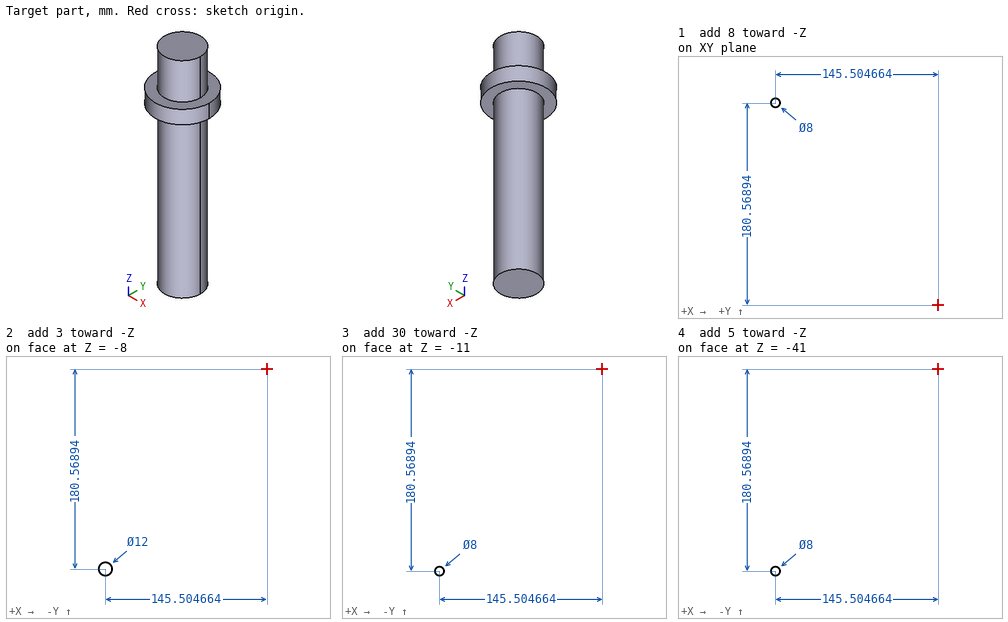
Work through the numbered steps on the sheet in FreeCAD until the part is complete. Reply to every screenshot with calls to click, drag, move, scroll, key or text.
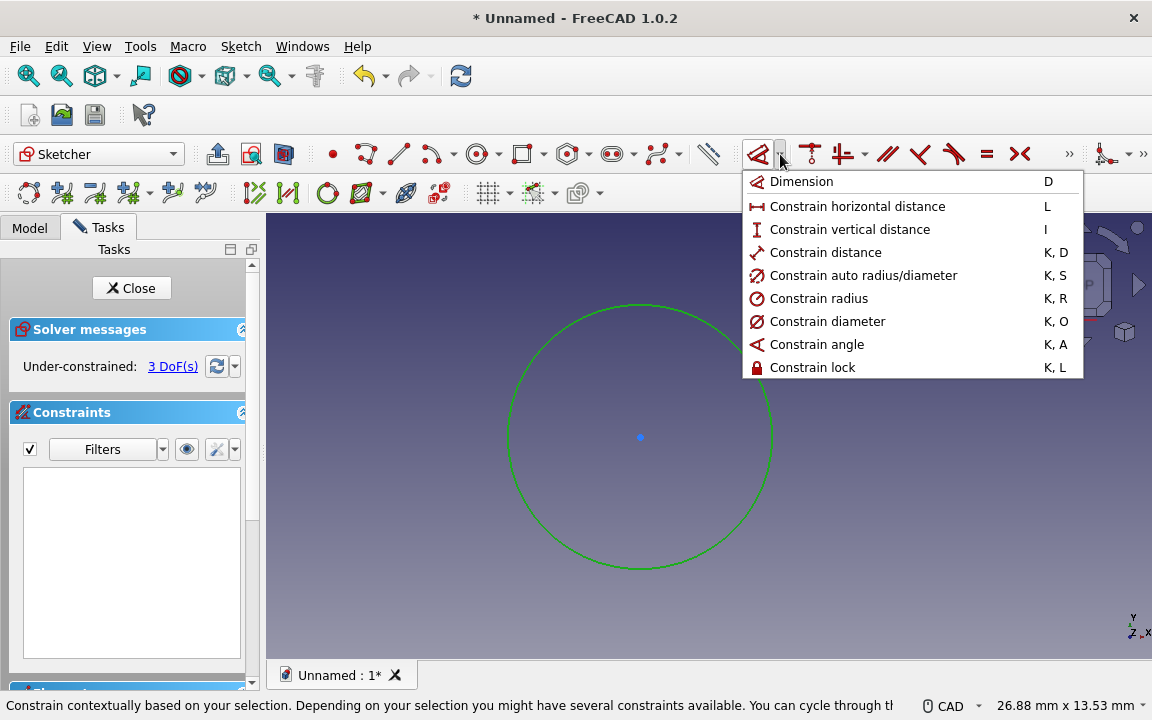
click(913, 322)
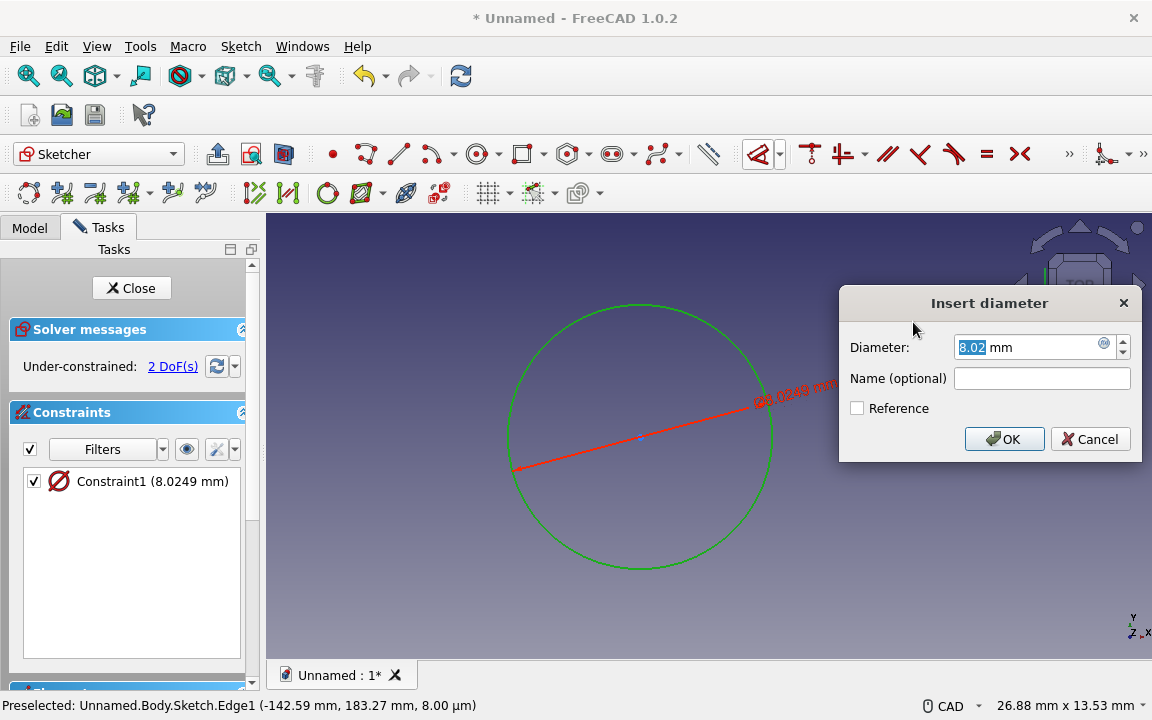
text(8)
key(Return)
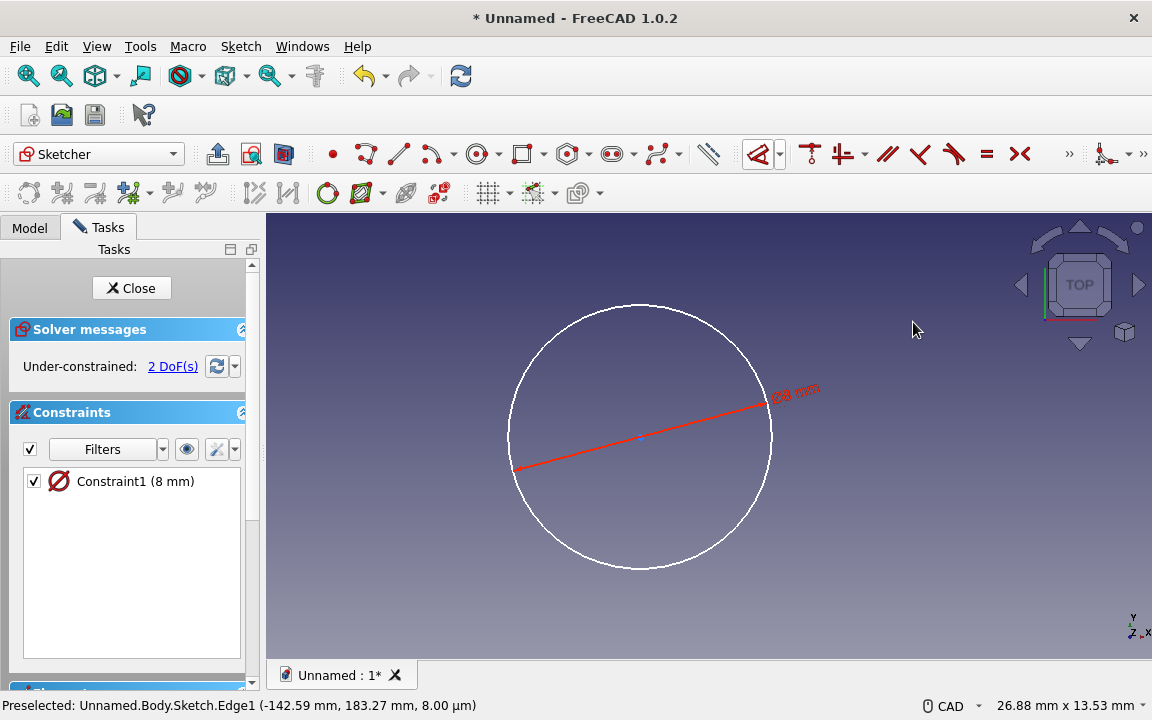
click(640, 437)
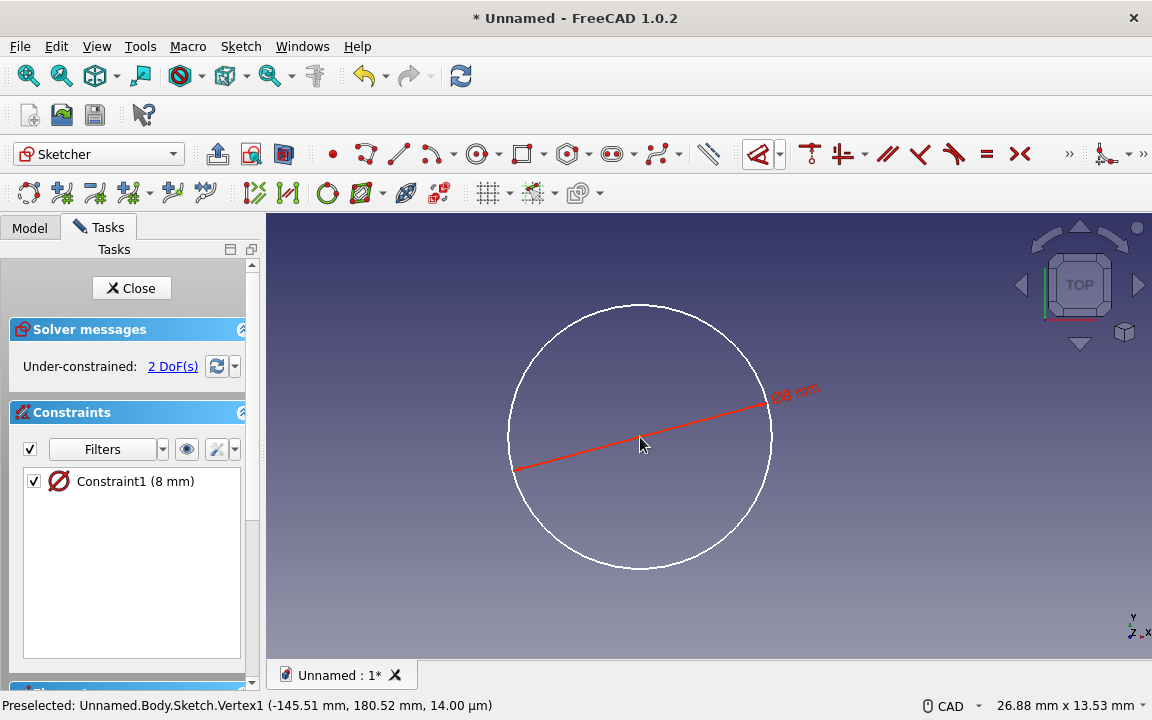
key(i)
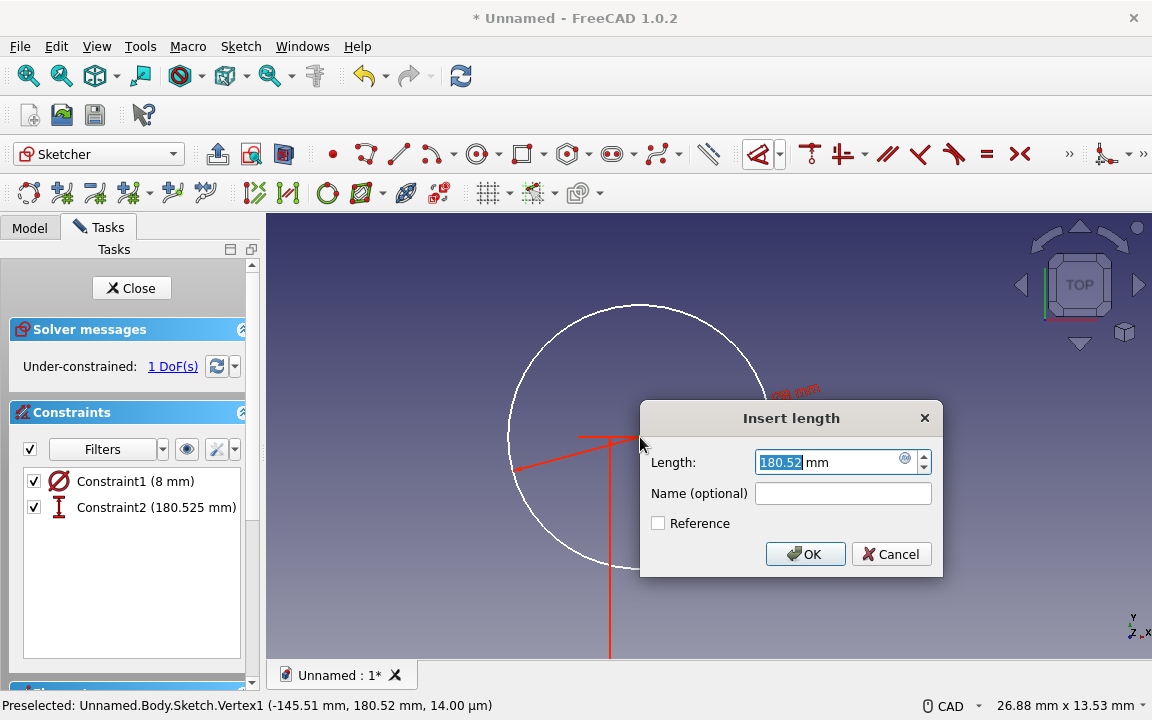
text(180.56894)
key(Return)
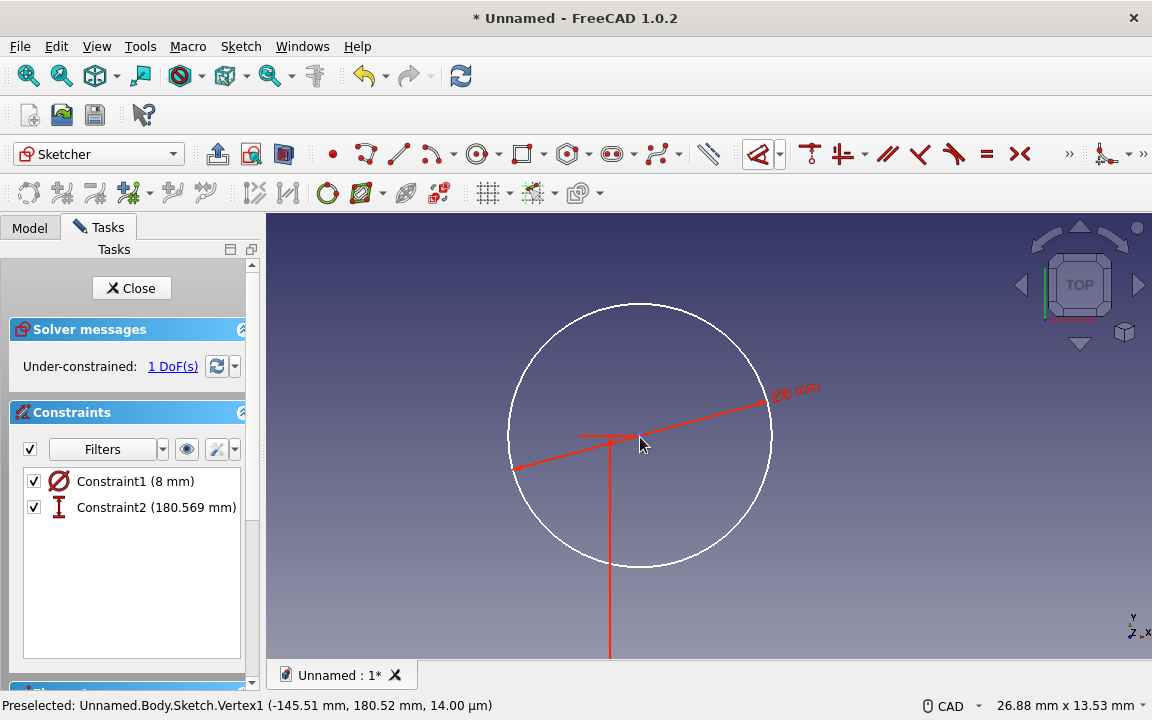
click(640, 436)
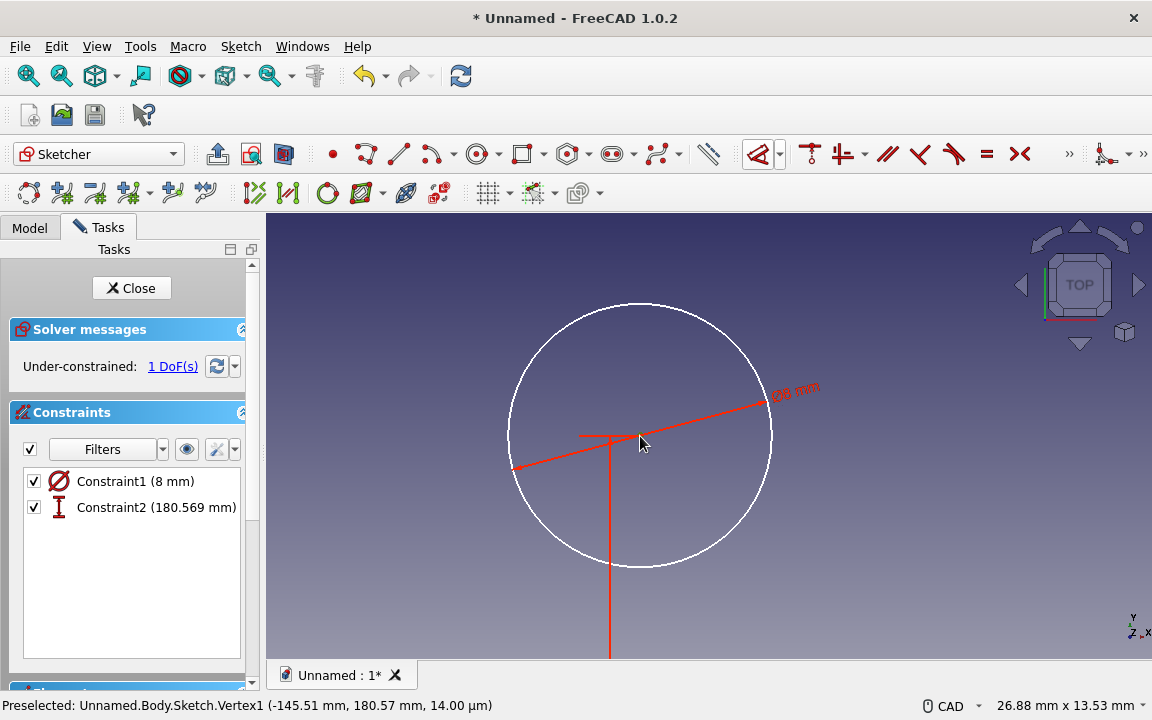
key(l)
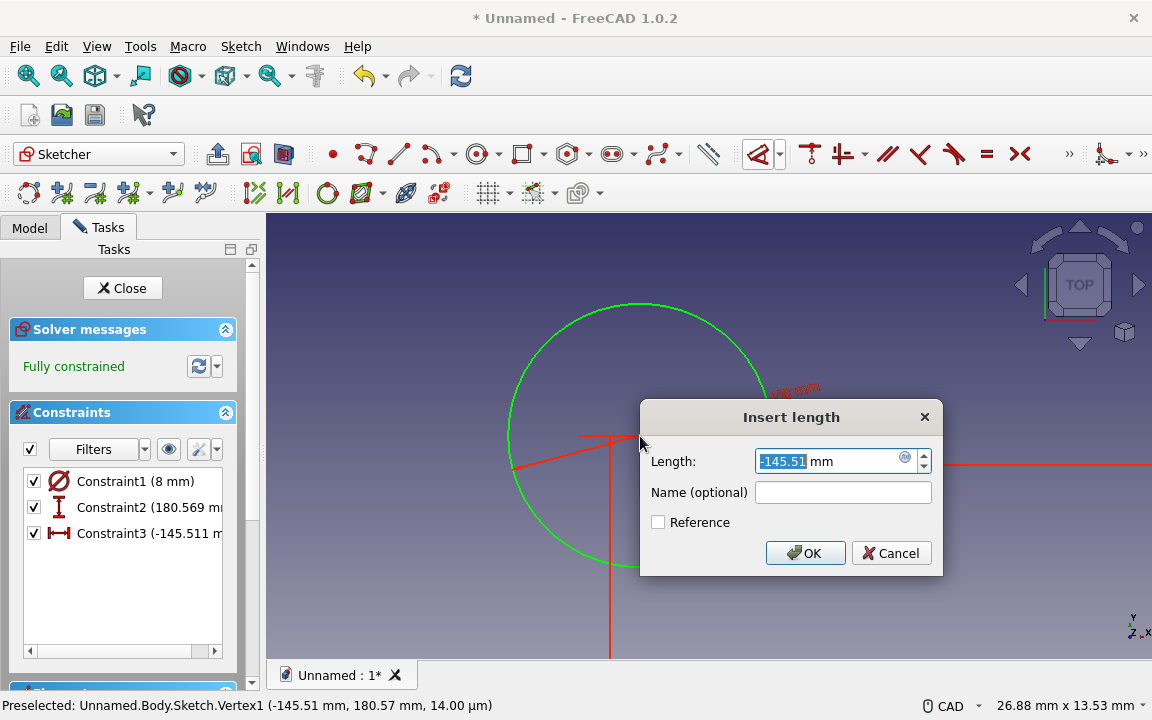
text(-145.504664)
key(Return)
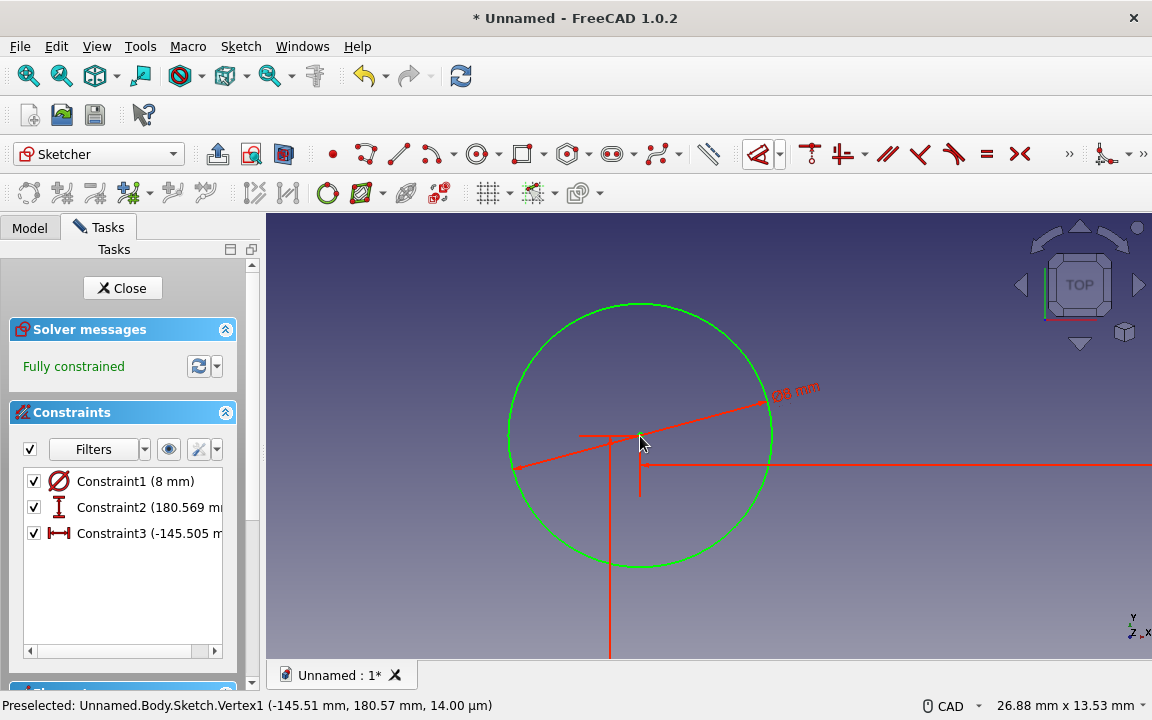
click(123, 288)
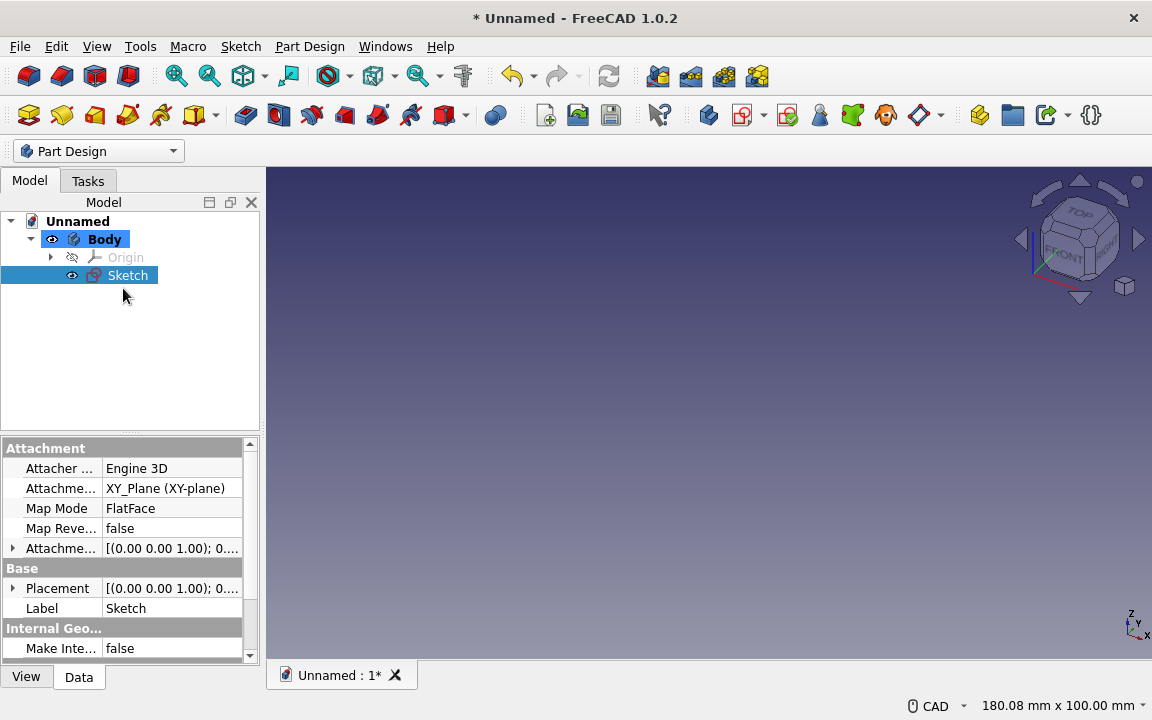
click(29, 116)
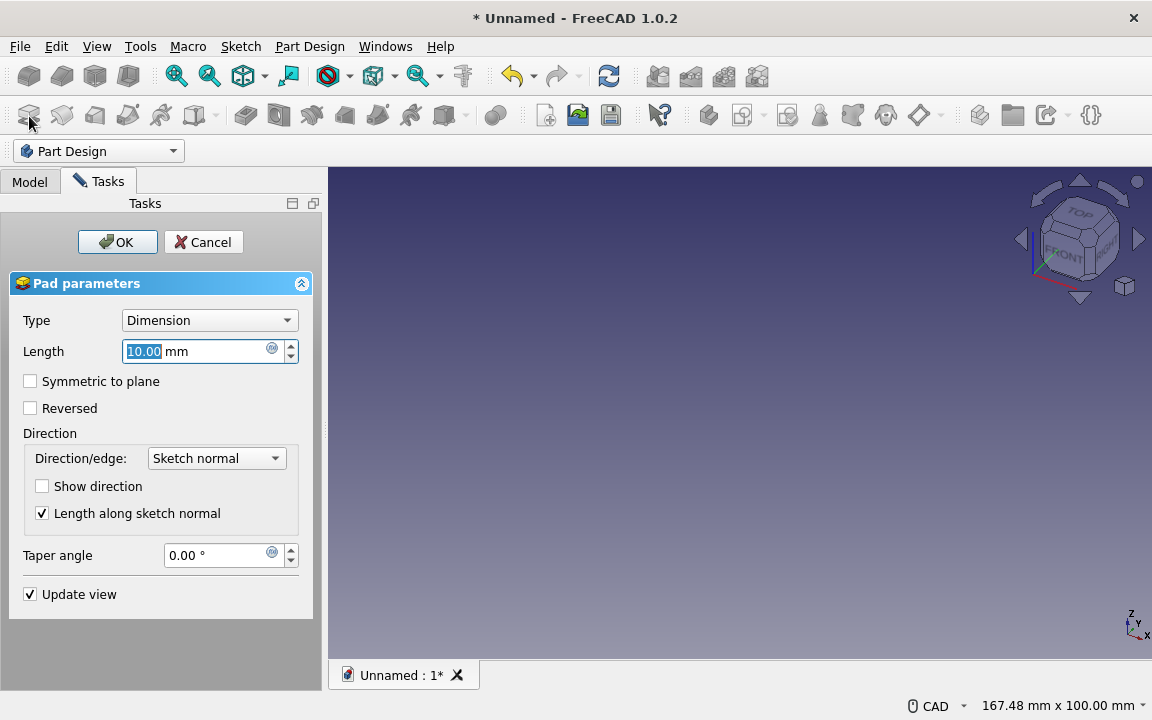
text(8)
key(Tab)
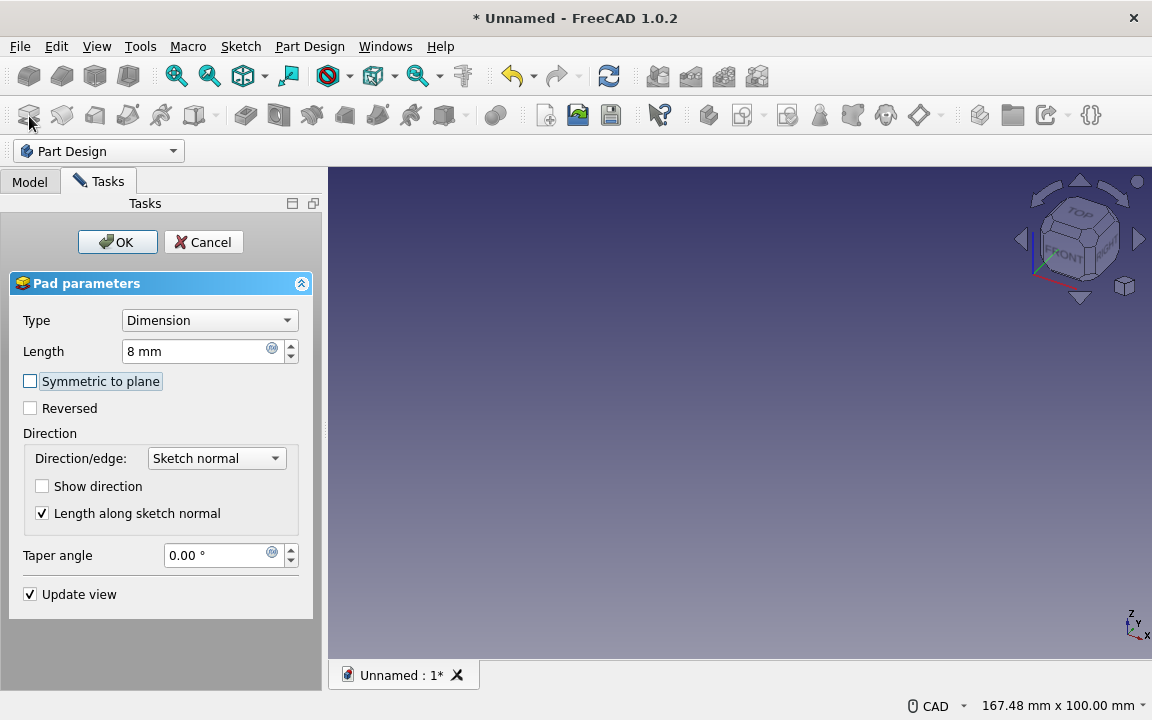
click(31, 408)